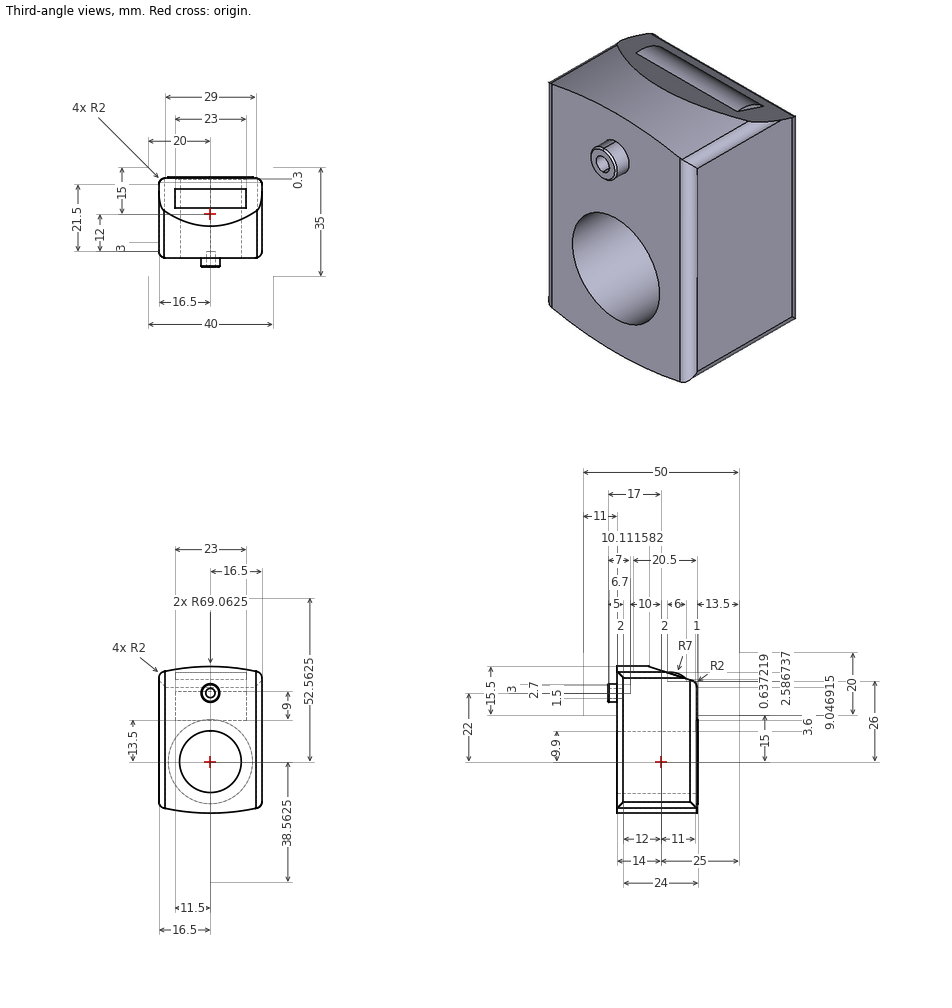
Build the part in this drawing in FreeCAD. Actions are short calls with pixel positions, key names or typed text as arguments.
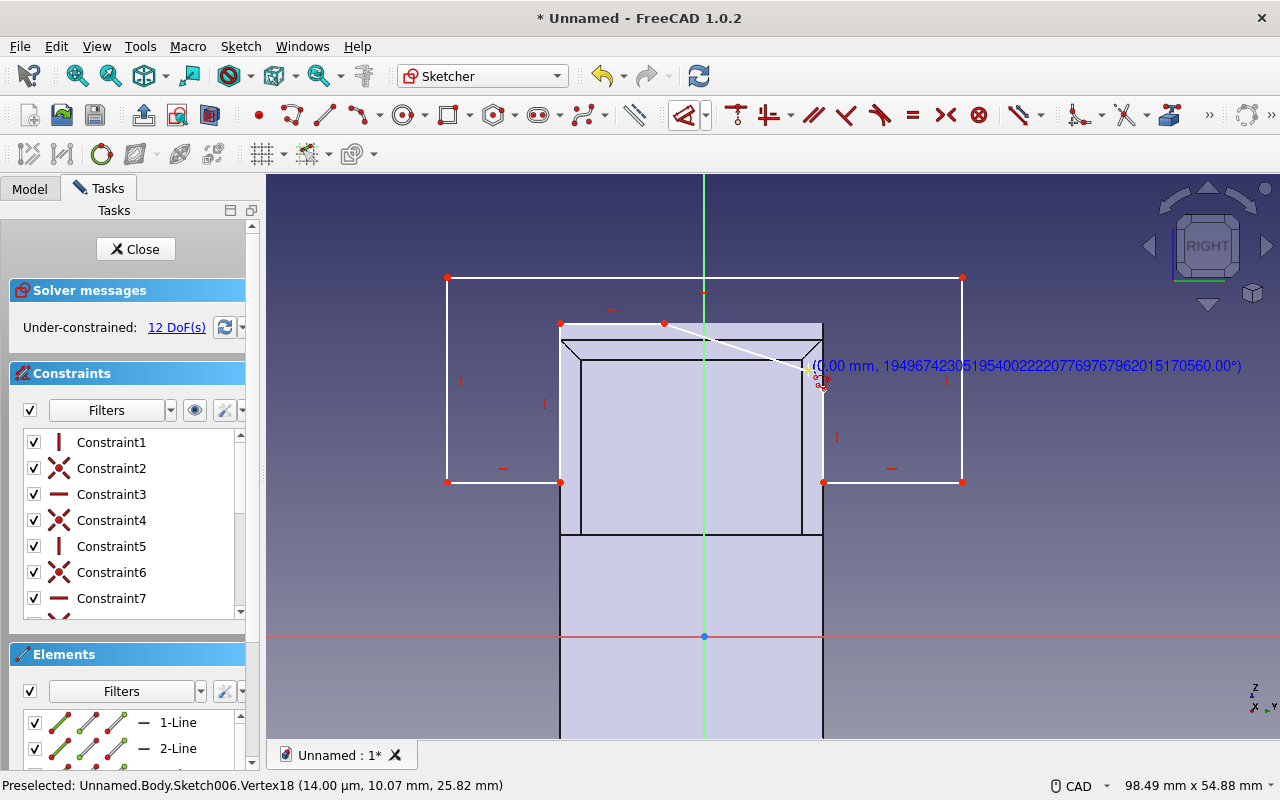
click(358, 116)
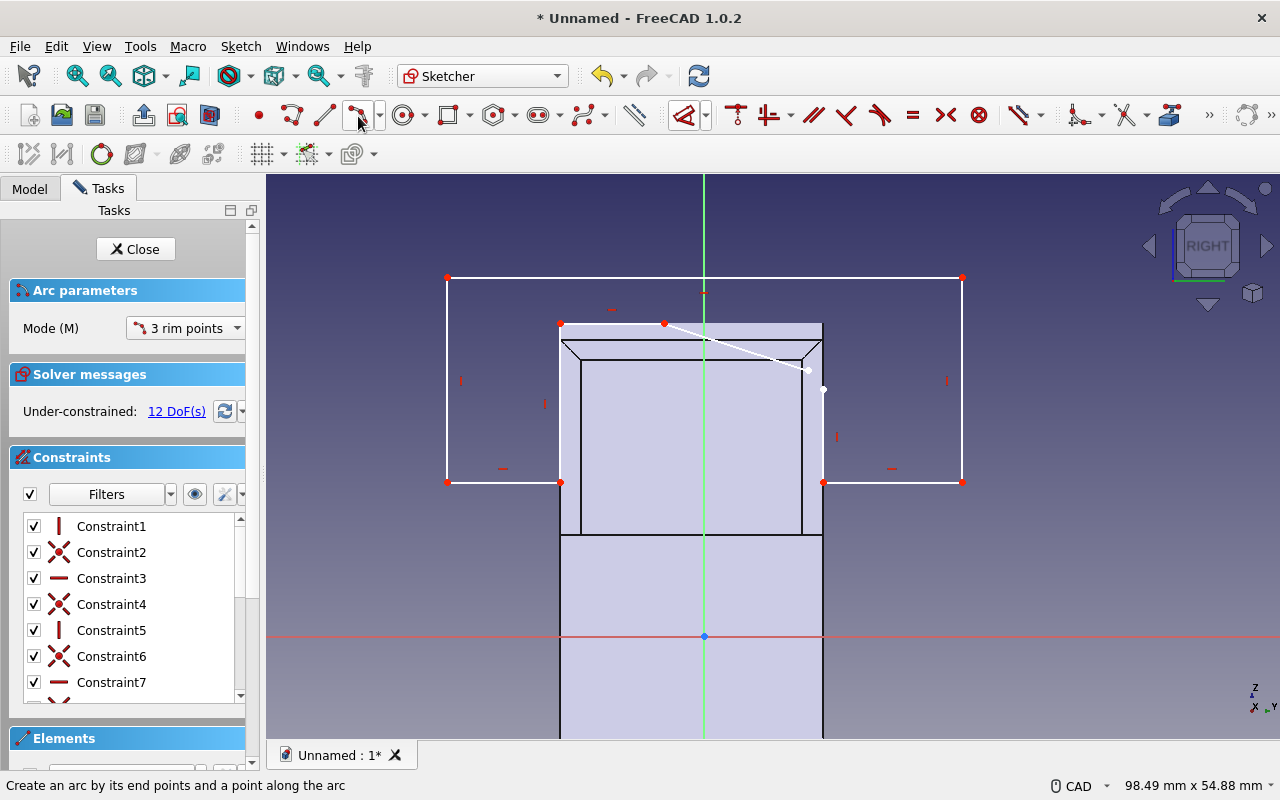
click(808, 371)
click(823, 390)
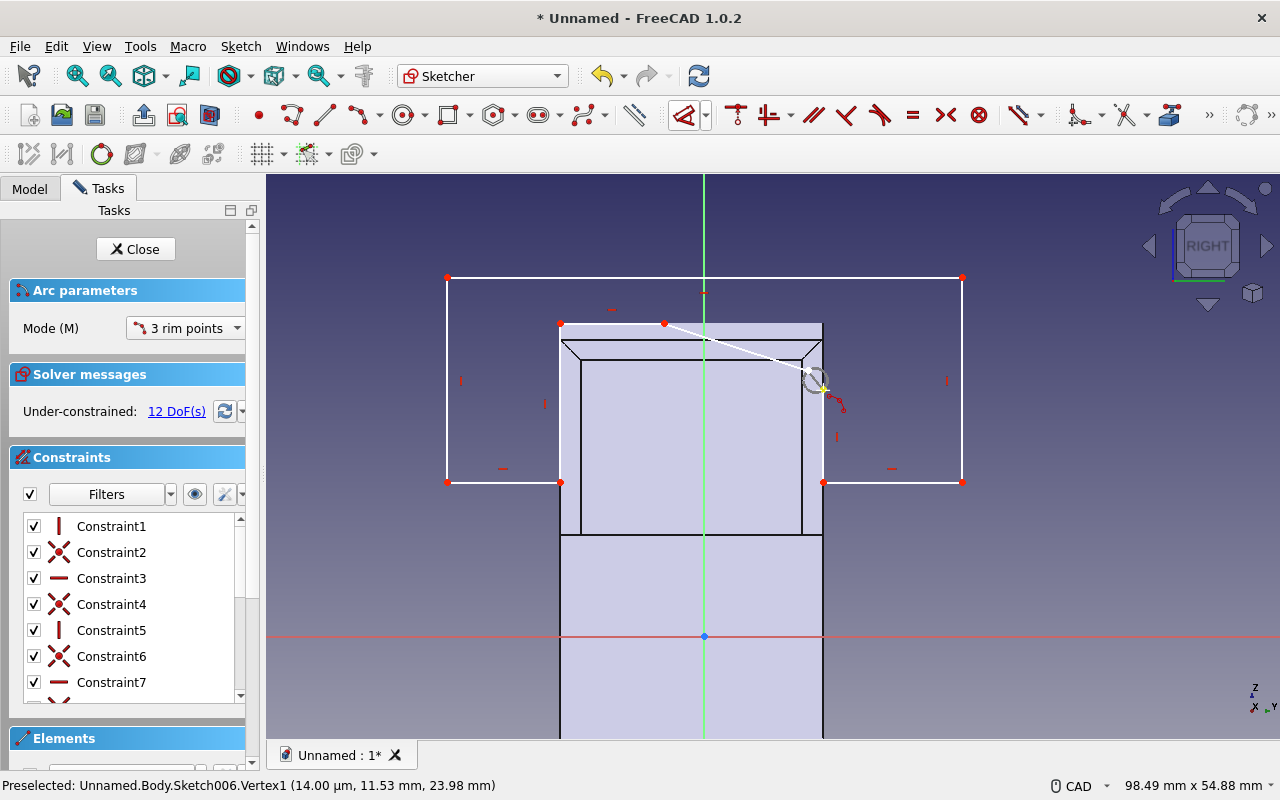
scroll(819, 377, up, 7)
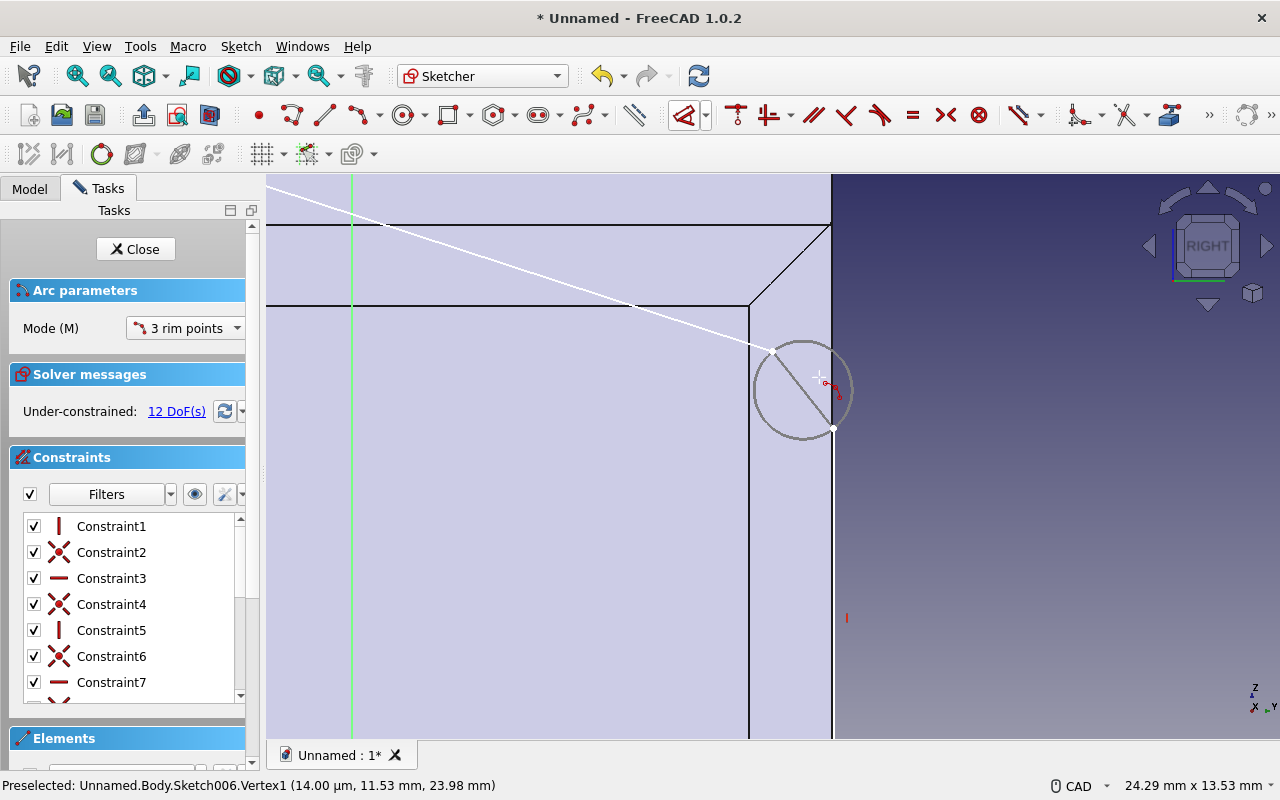
click(816, 377)
key(Escape)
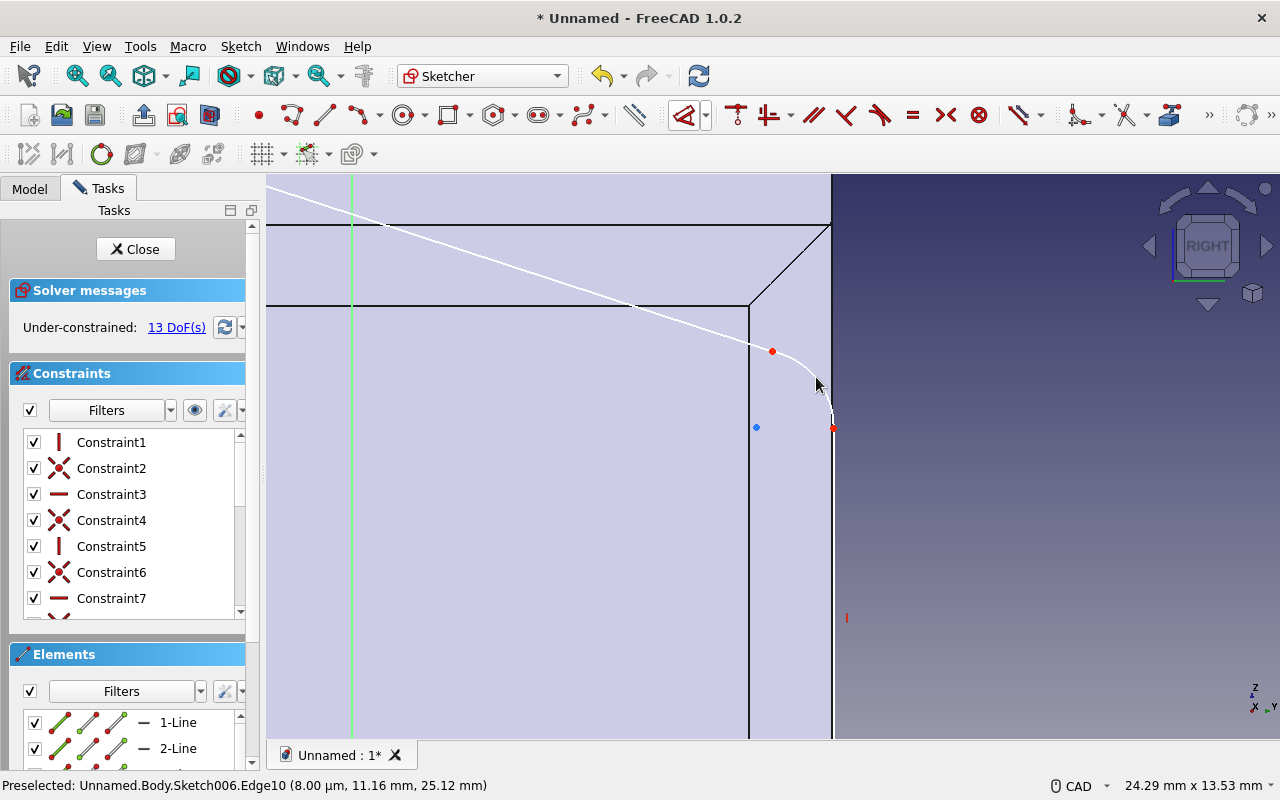
scroll(820, 377, down, 7)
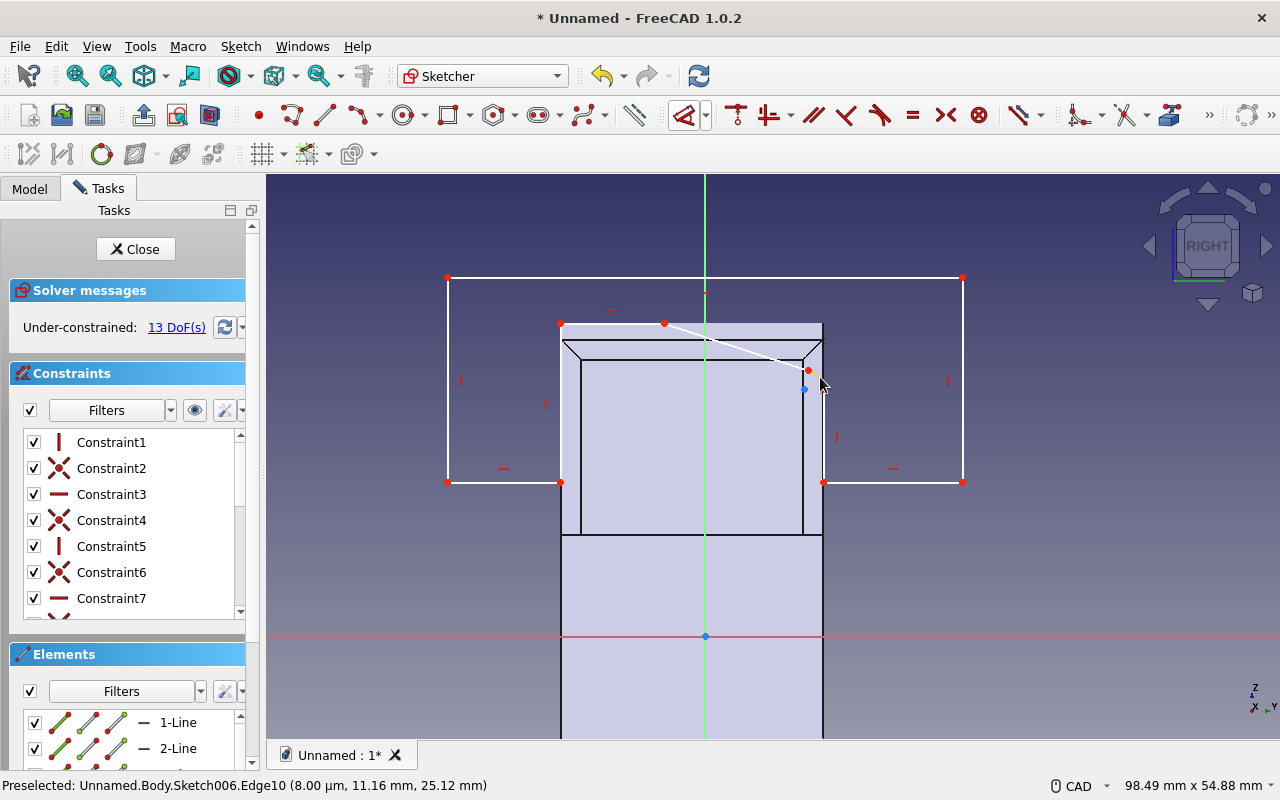
click(824, 418)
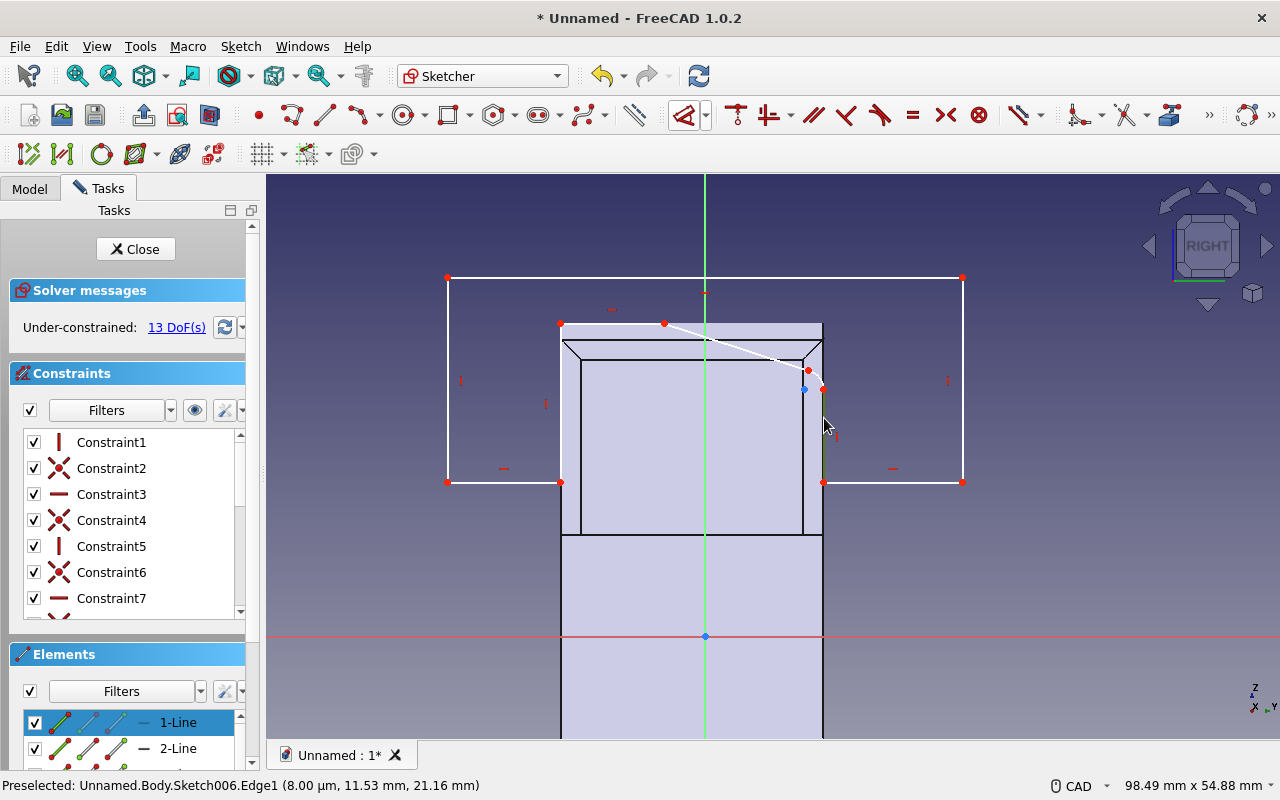
click(820, 378)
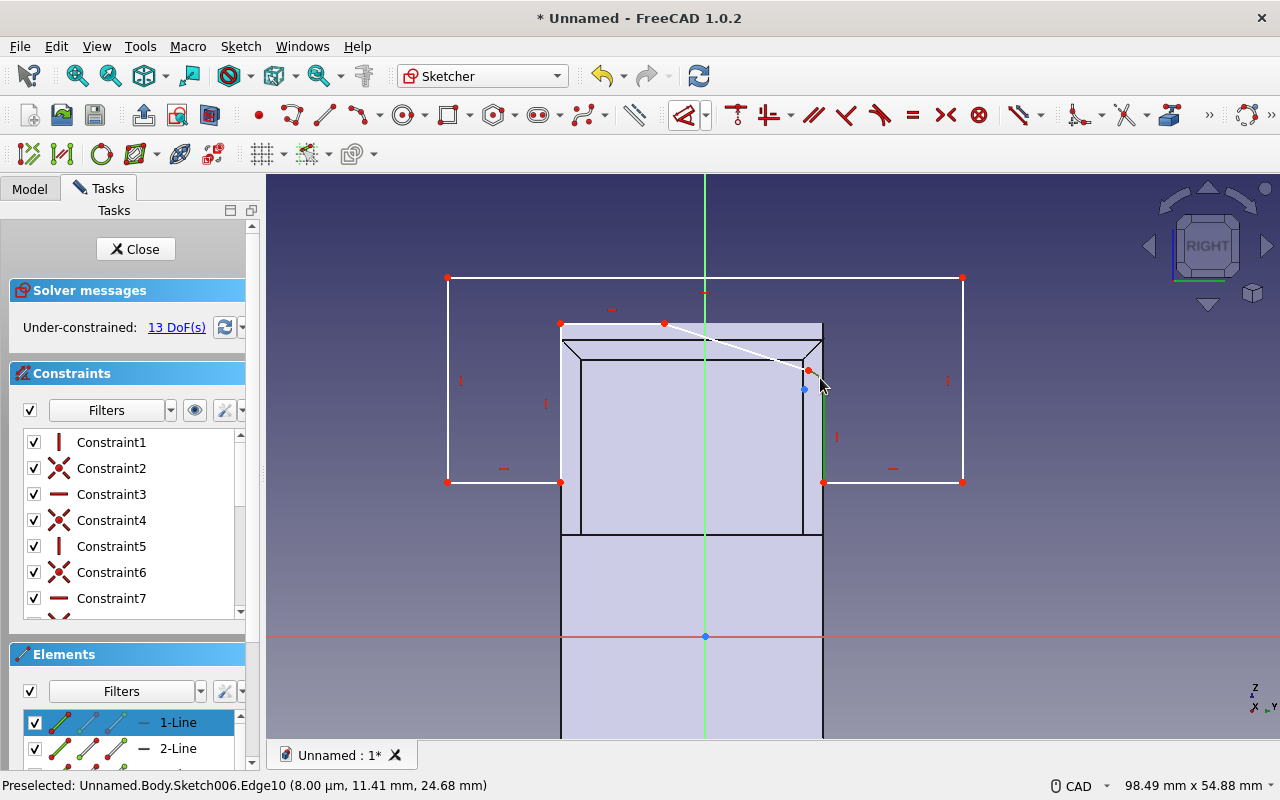
click(880, 116)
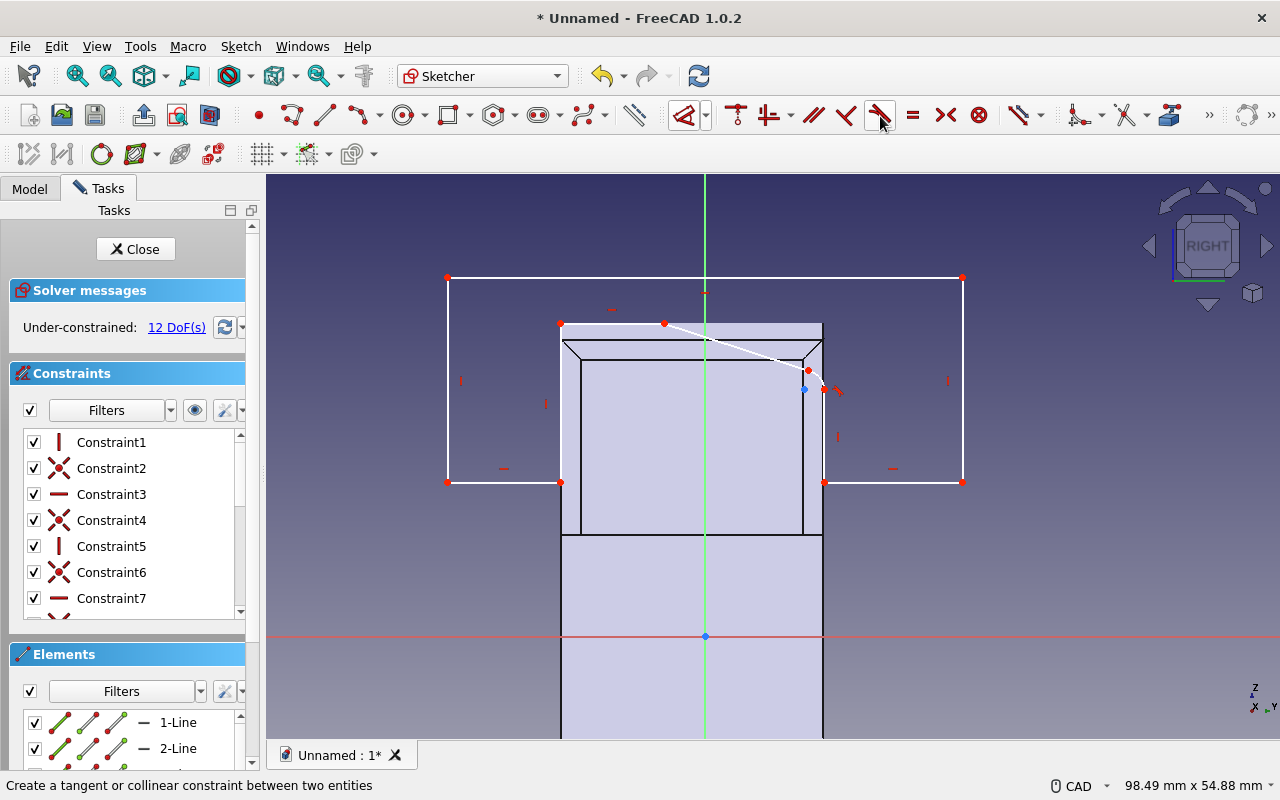
click(708, 338)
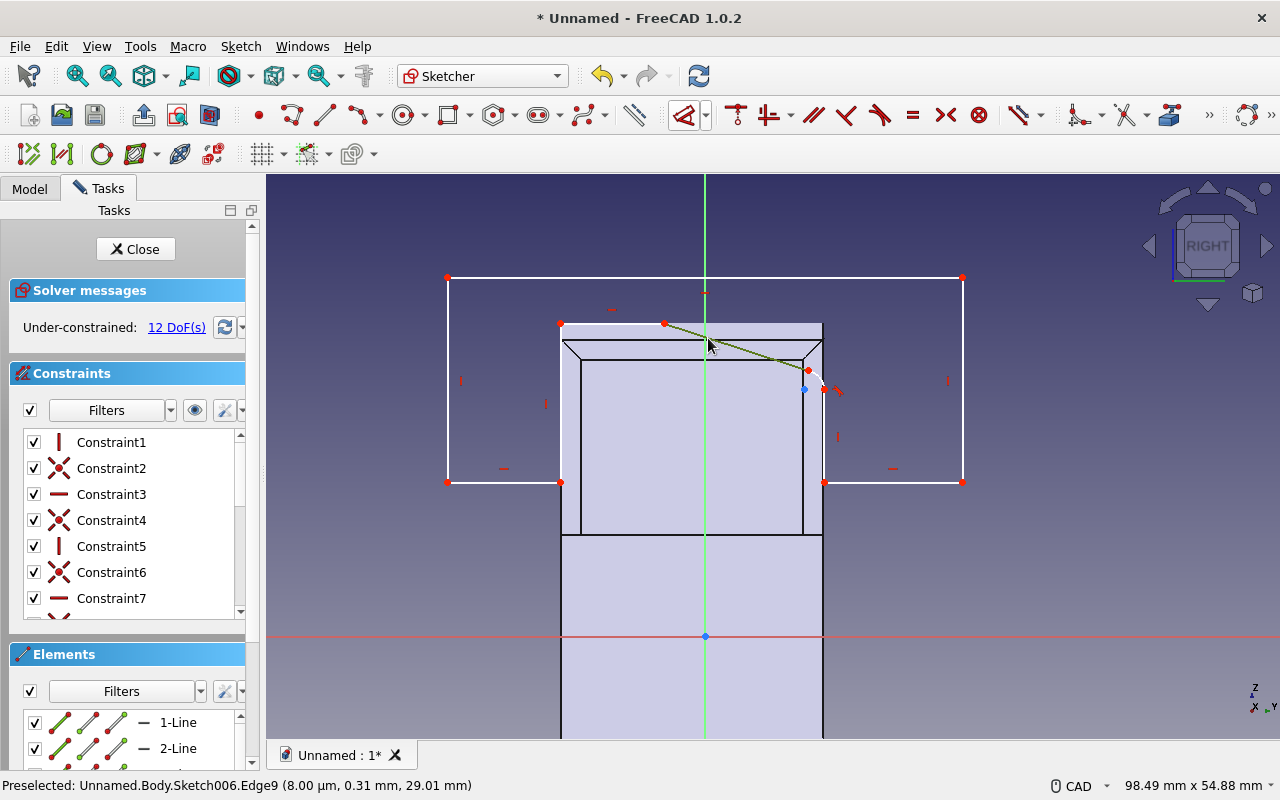
click(820, 378)